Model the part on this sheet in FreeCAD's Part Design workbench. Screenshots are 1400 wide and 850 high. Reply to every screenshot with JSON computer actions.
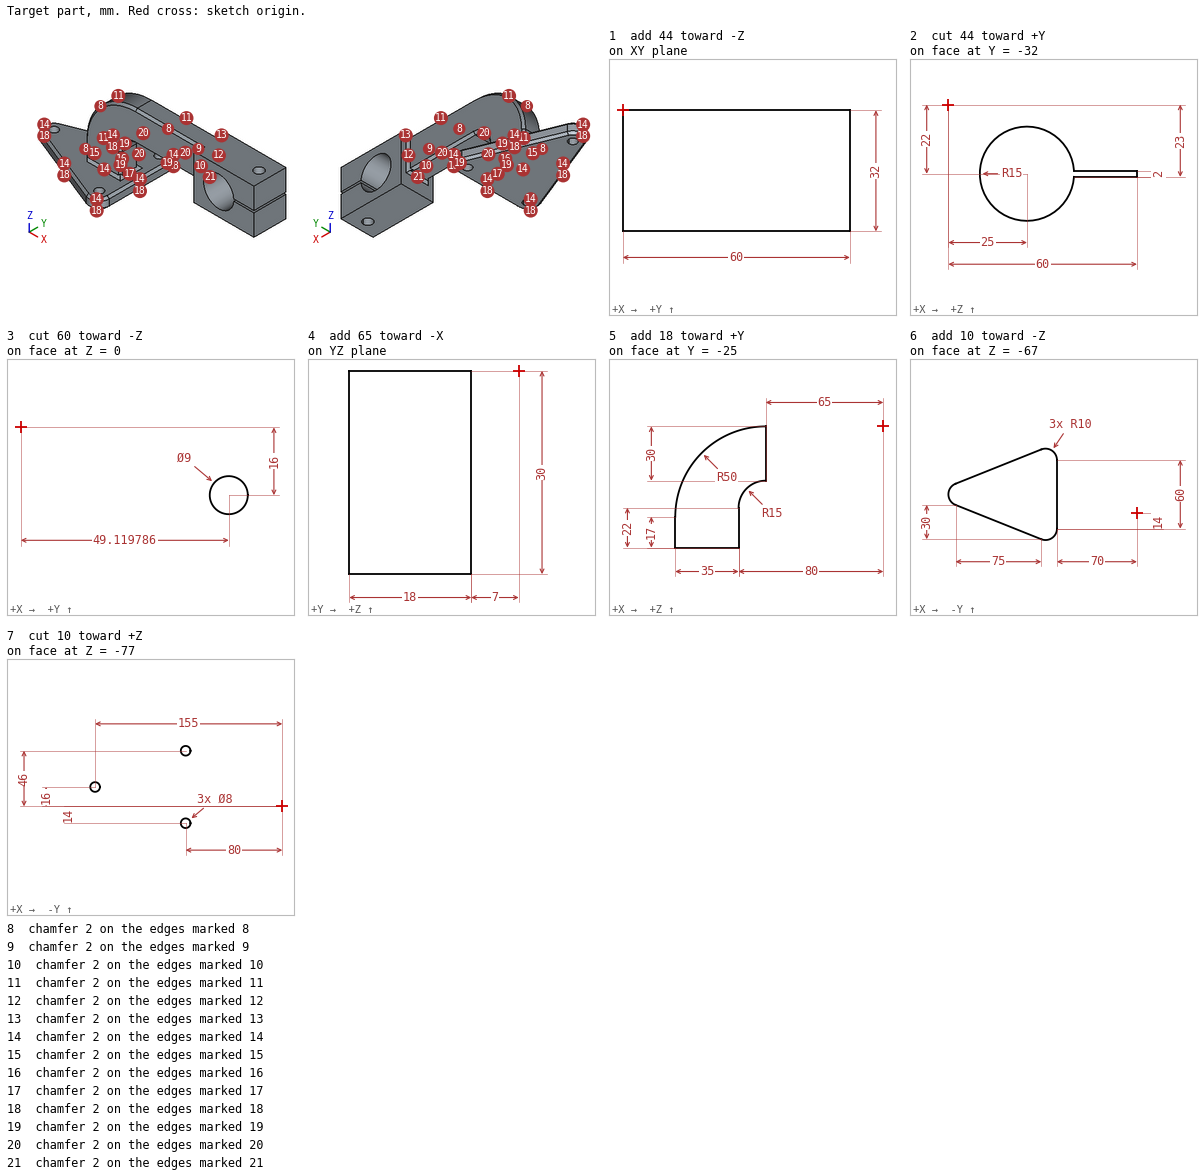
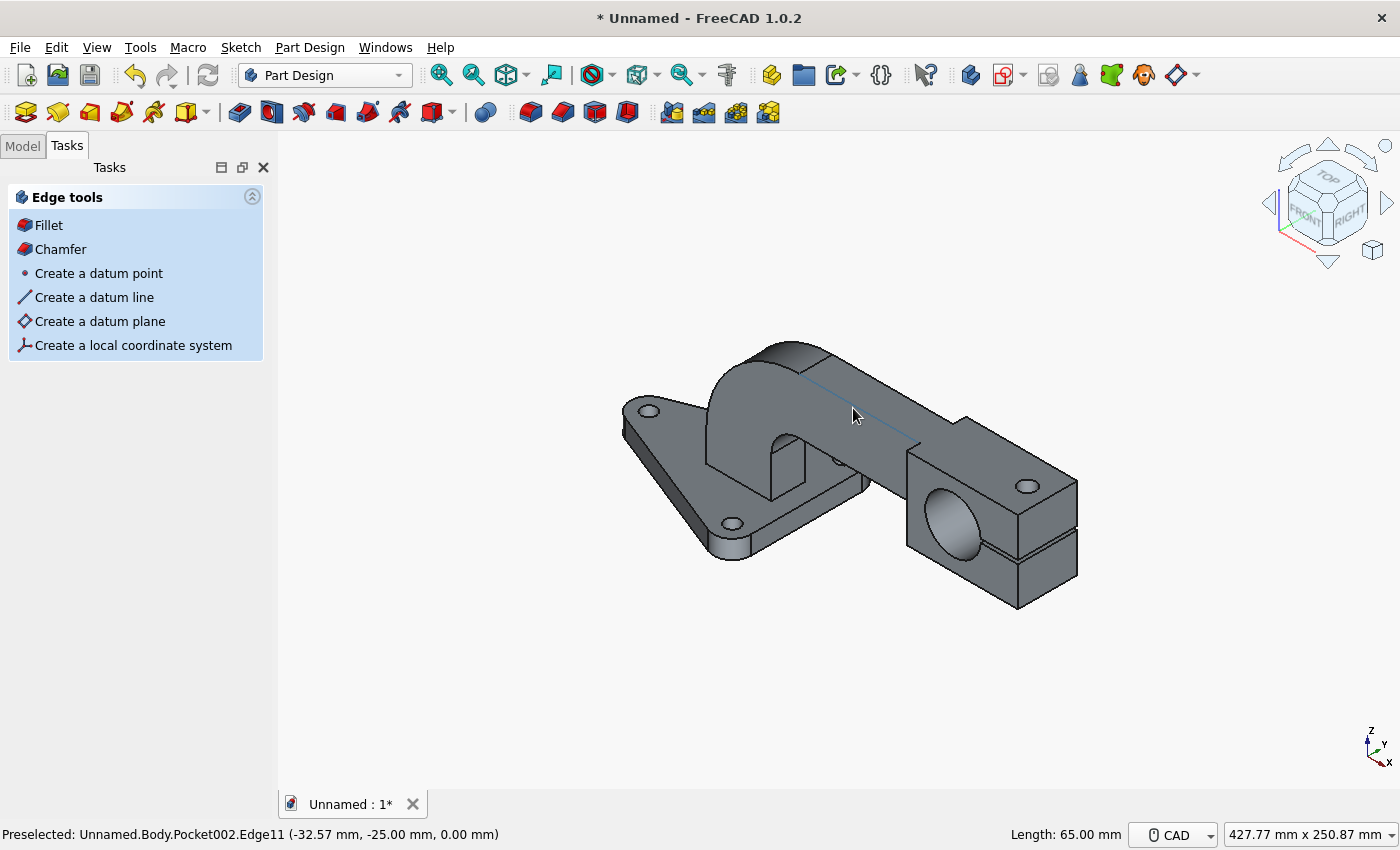
{"action": "left_click", "coordinate": [734, 366], "text": "ctrl"}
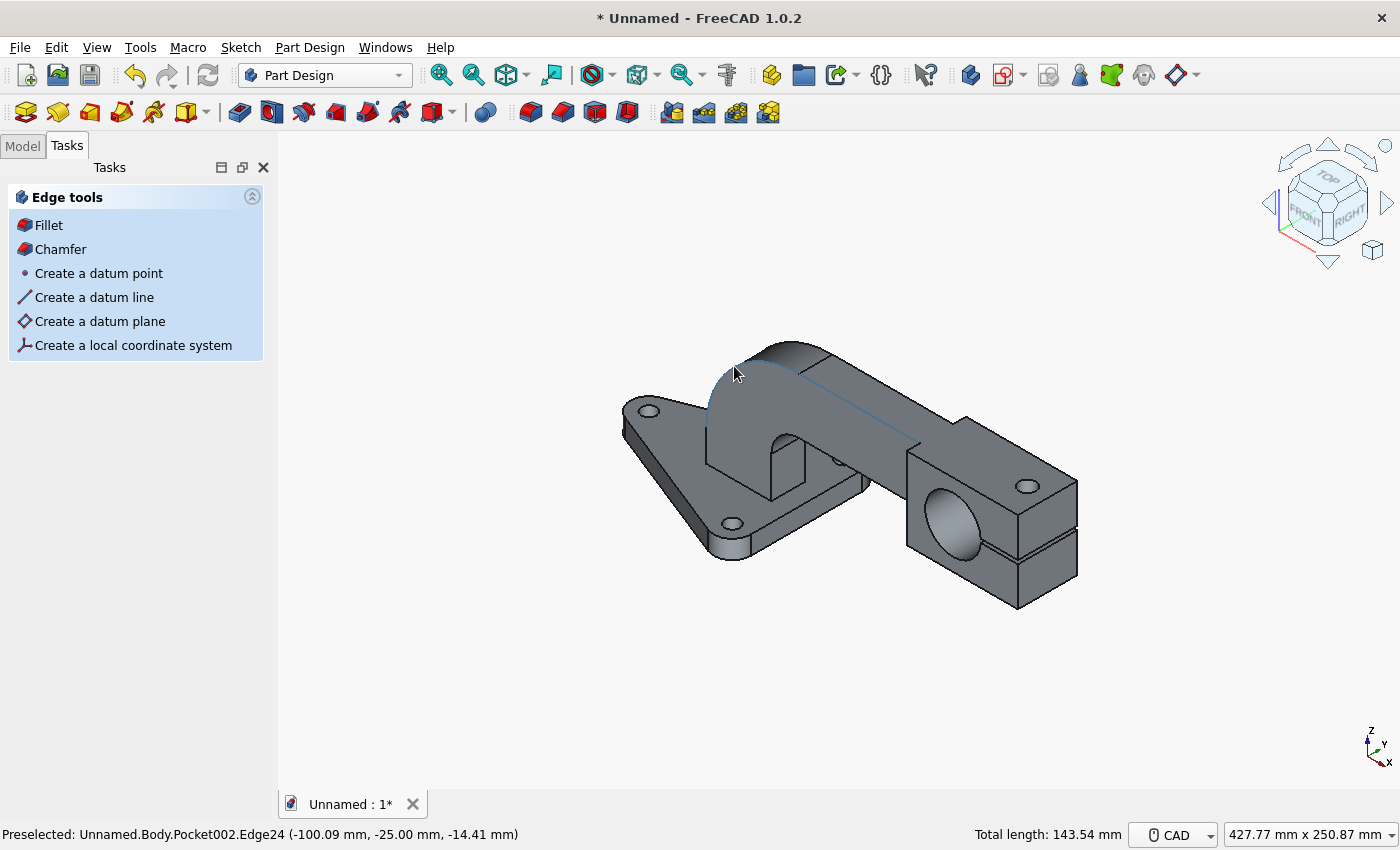
{"action": "key", "text": "2"}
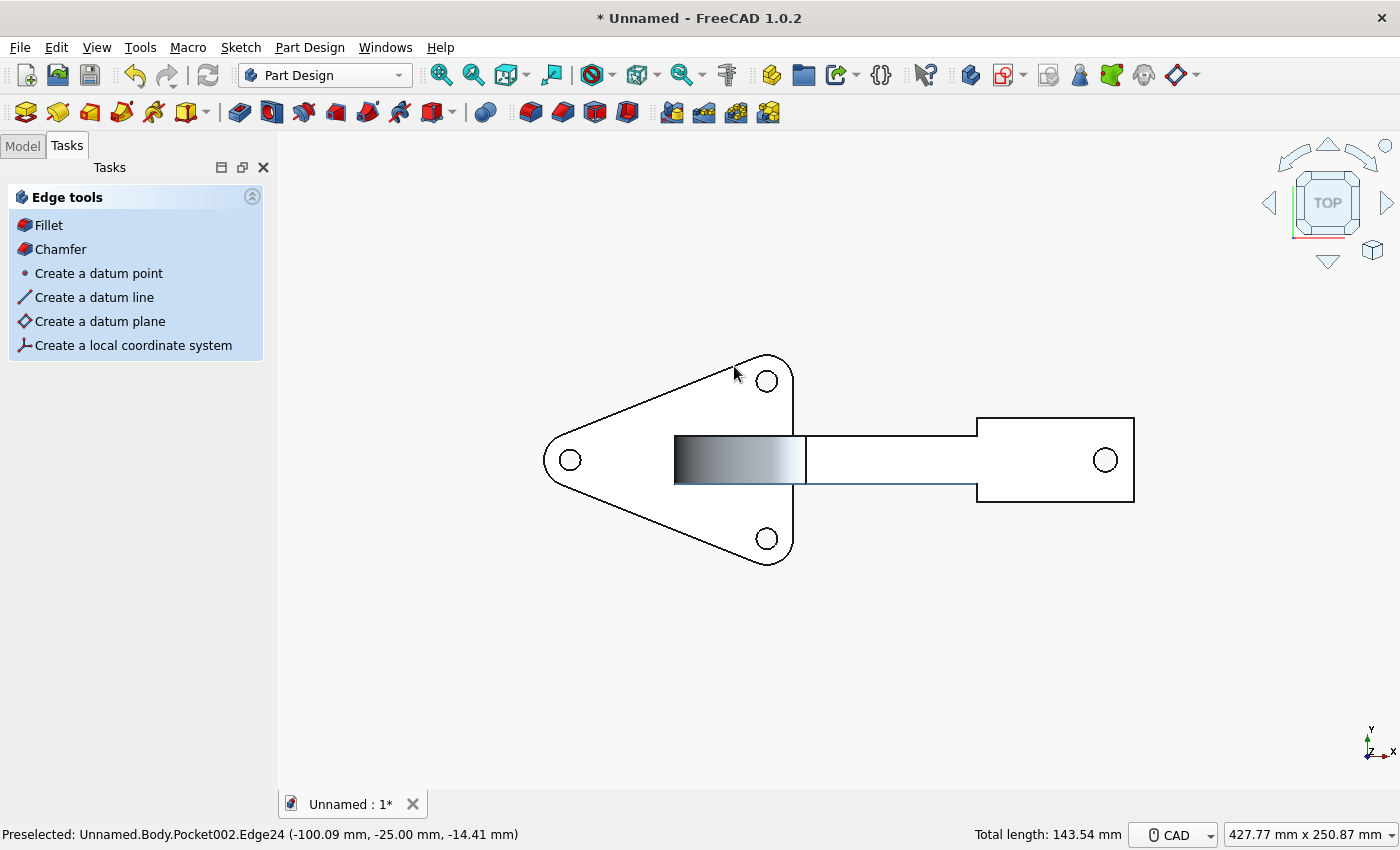
{"action": "key", "text": "1"}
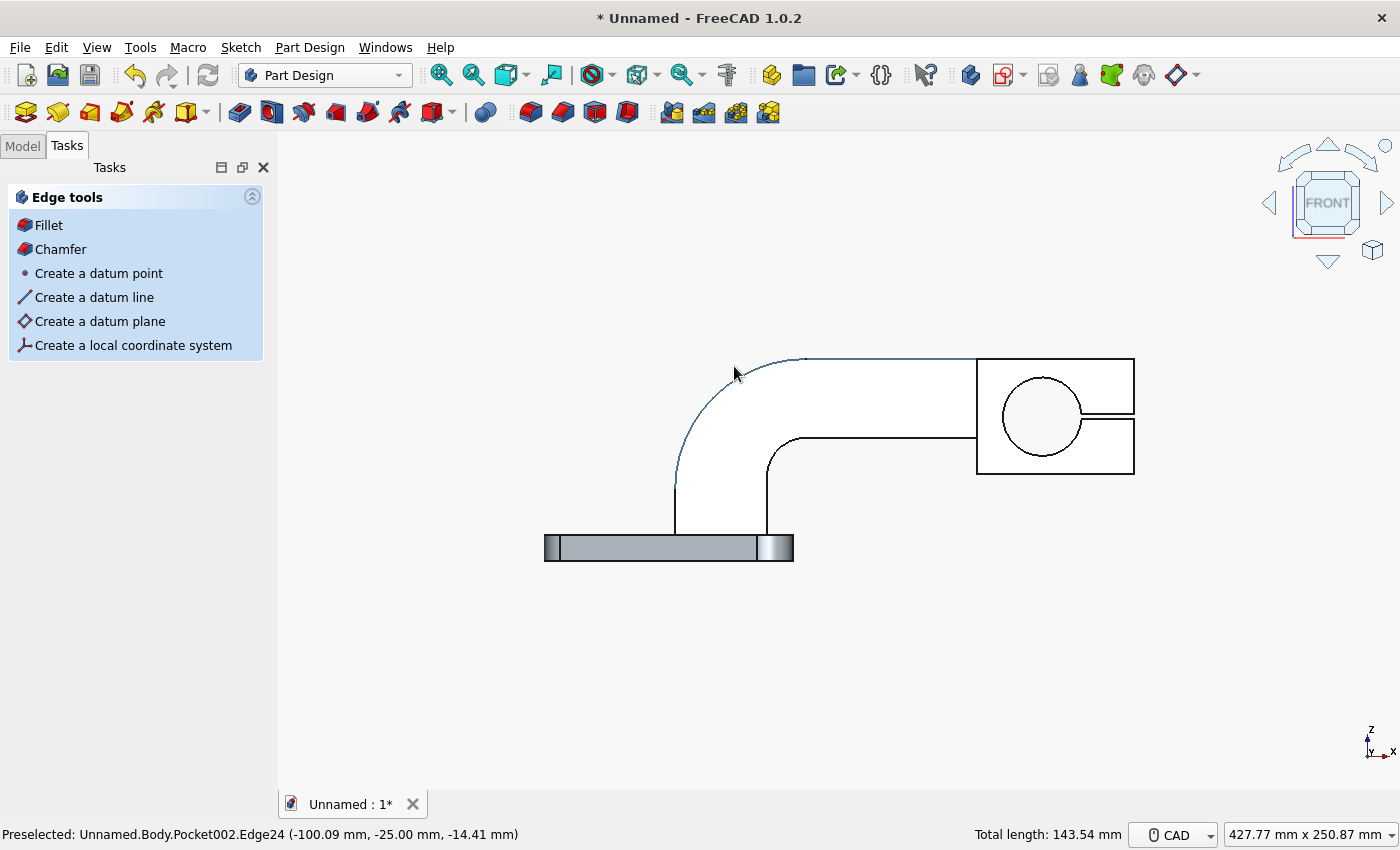
{"action": "left_click", "coordinate": [675, 511], "text": "ctrl"}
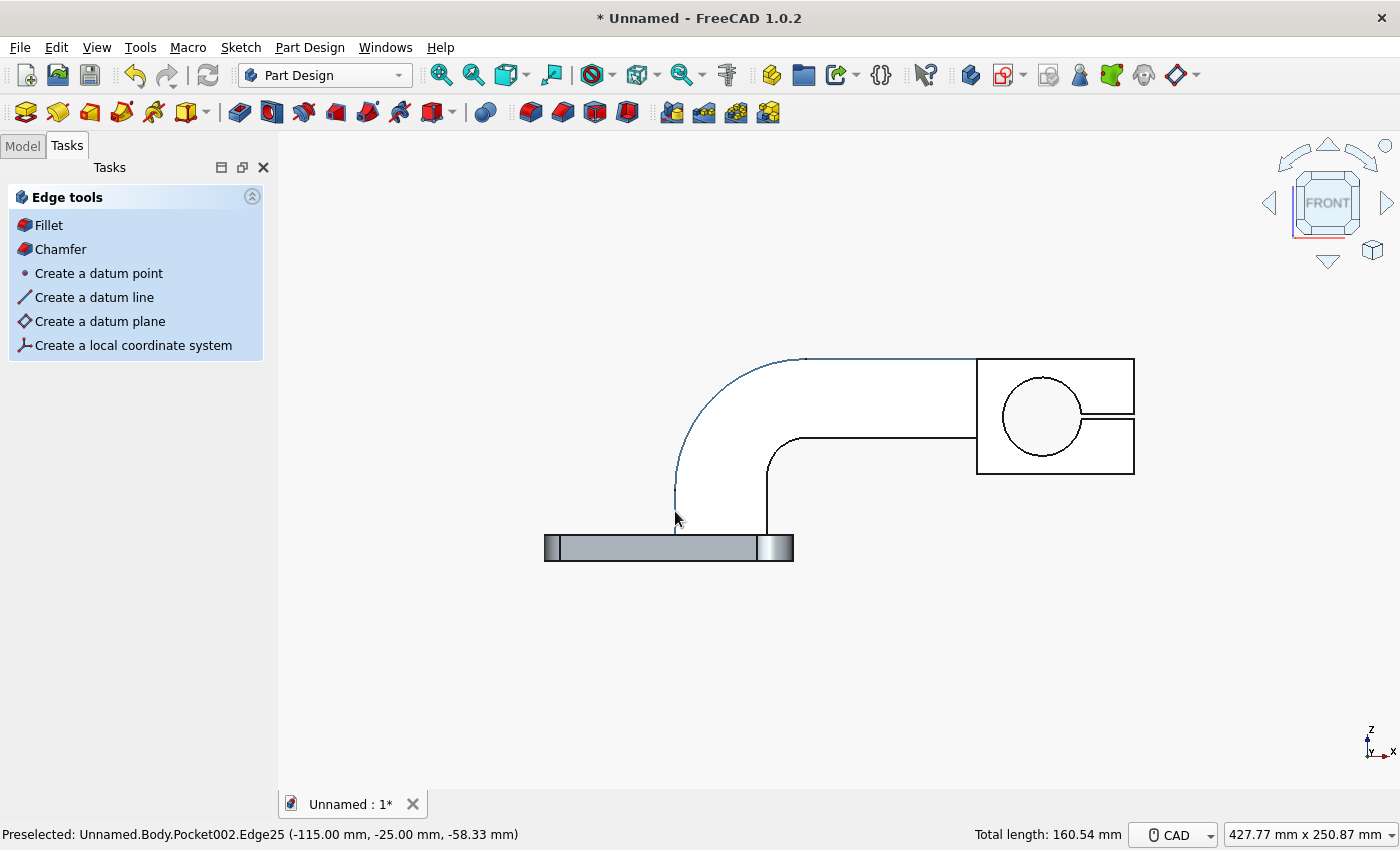
{"action": "left_click", "coordinate": [564, 112]}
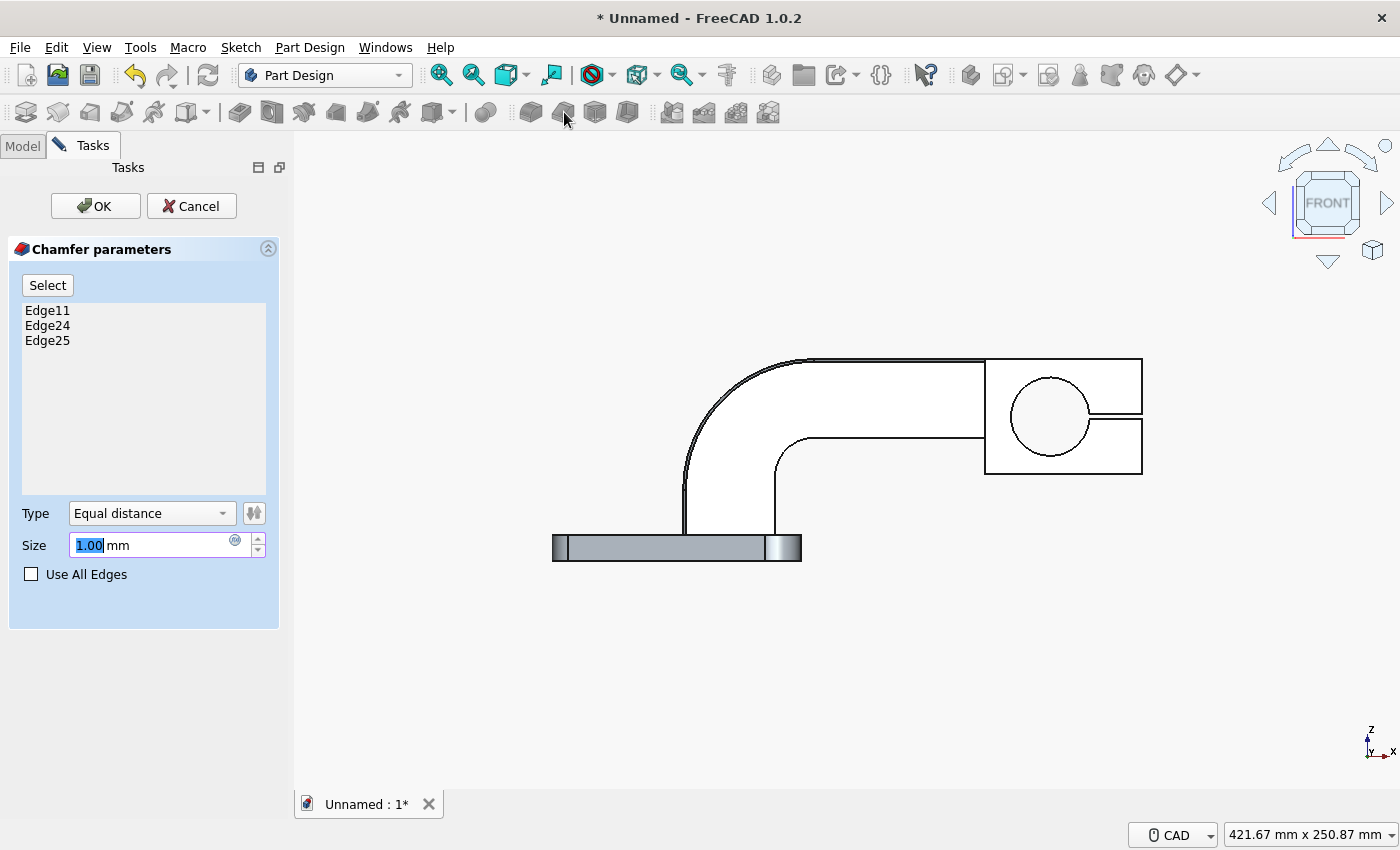
{"action": "type", "text": "2"}
{"action": "key", "text": "Tab"}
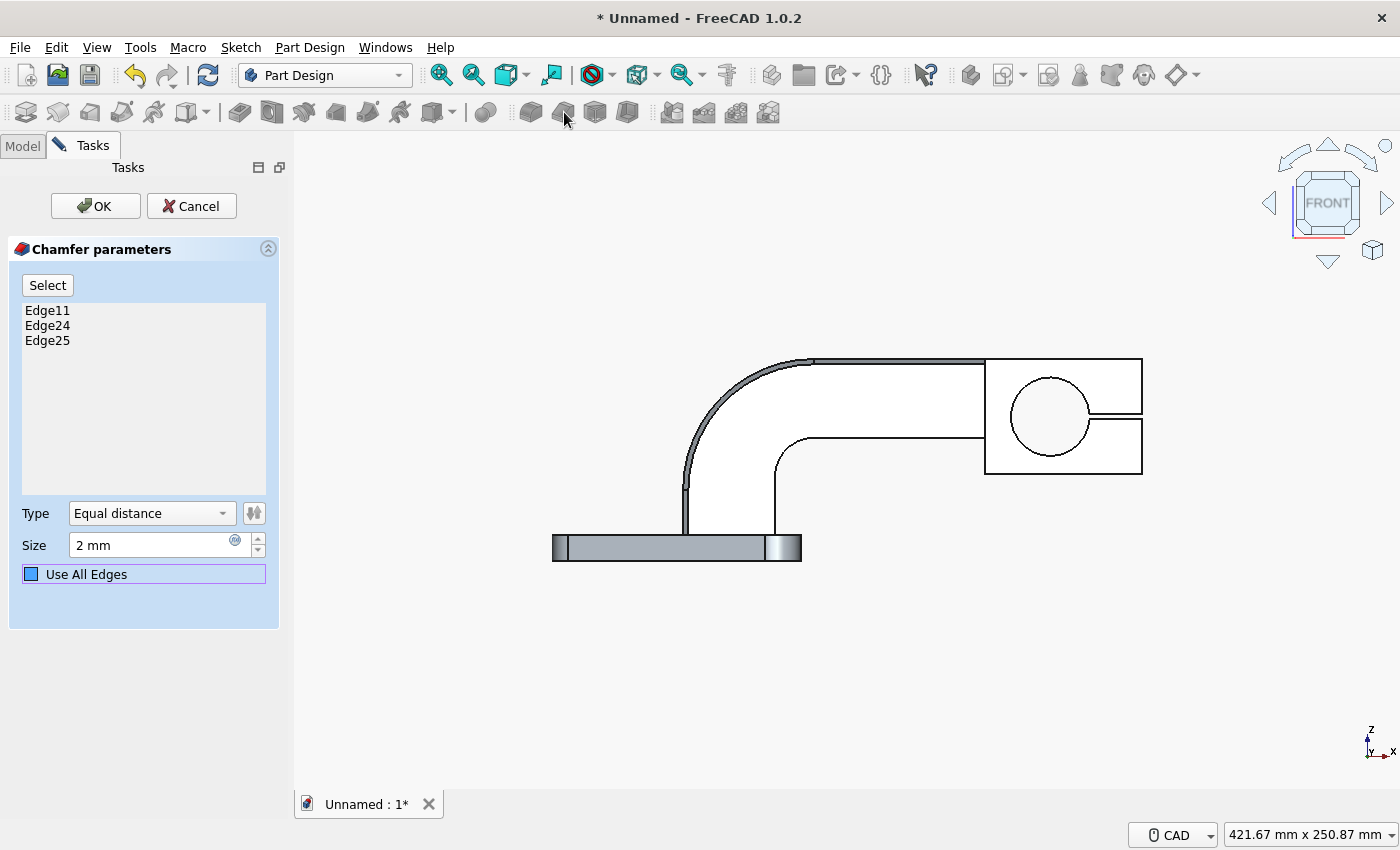
{"action": "left_click", "coordinate": [96, 206]}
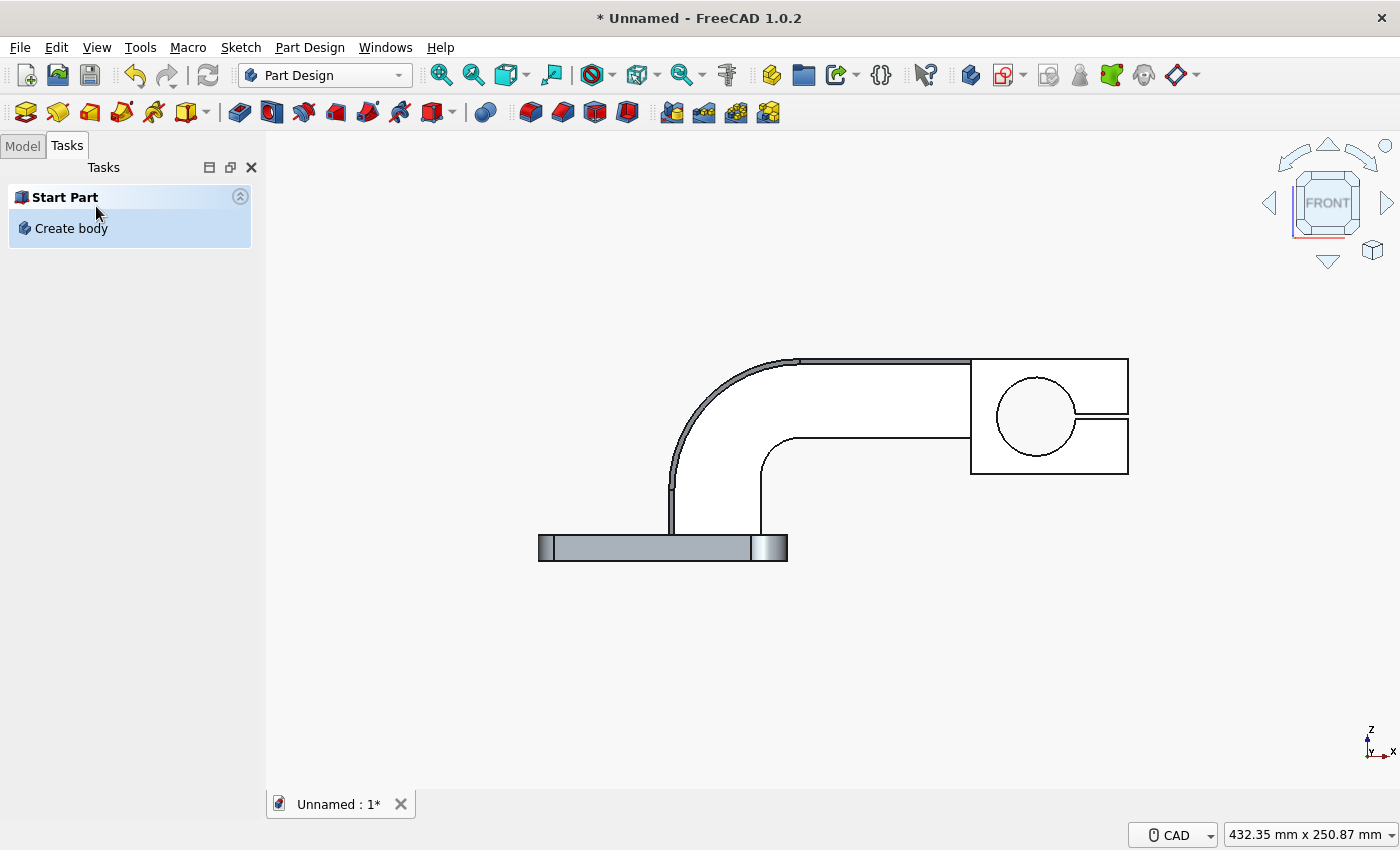
{"action": "scroll", "coordinate": [971, 358], "scroll_direction": "up", "scroll_amount": 4}